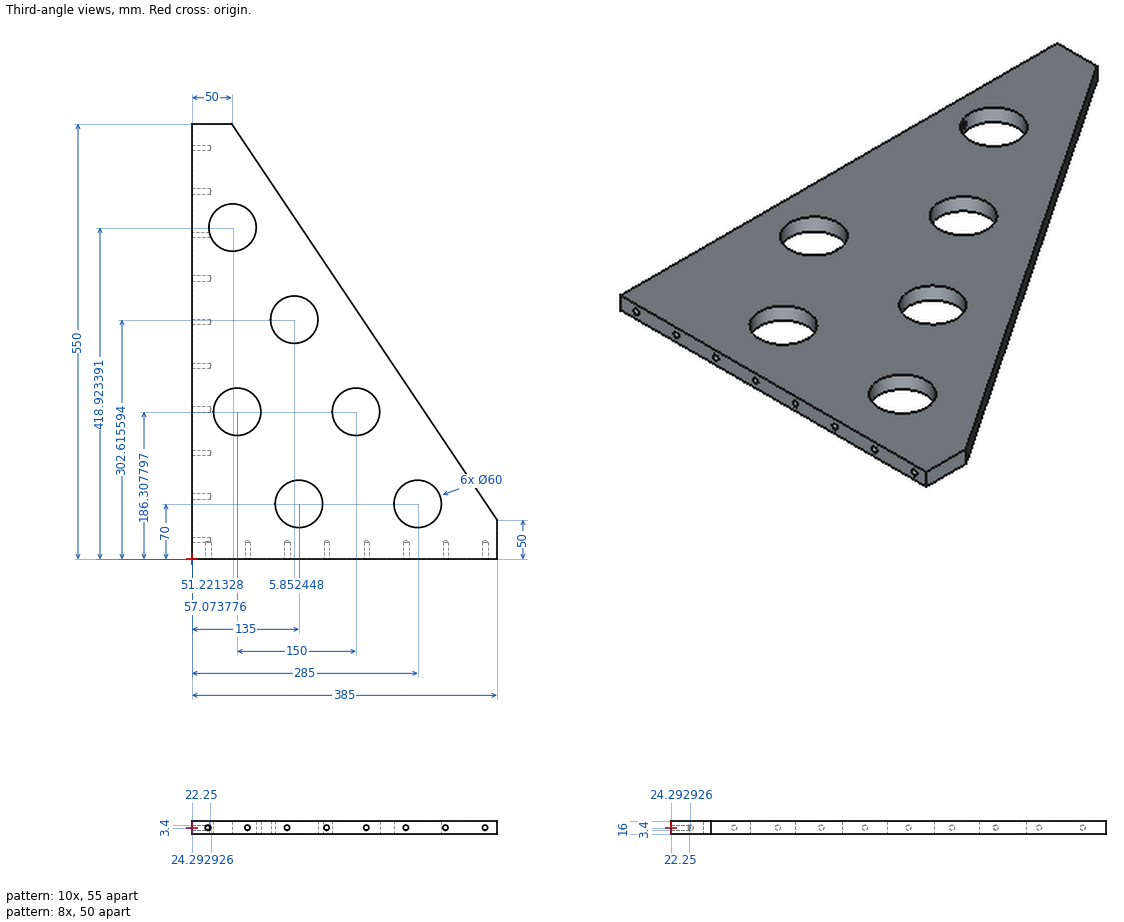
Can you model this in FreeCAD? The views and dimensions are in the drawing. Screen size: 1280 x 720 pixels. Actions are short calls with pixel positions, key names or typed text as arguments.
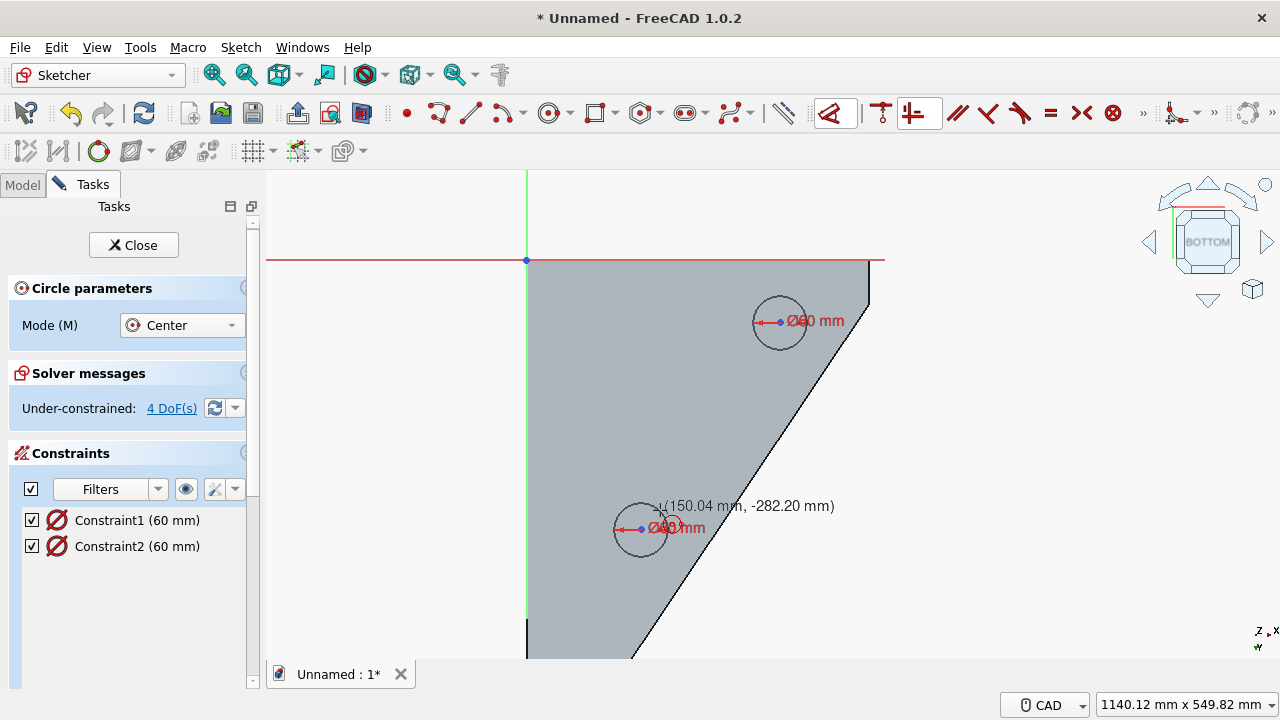
click(711, 426)
move(730, 407)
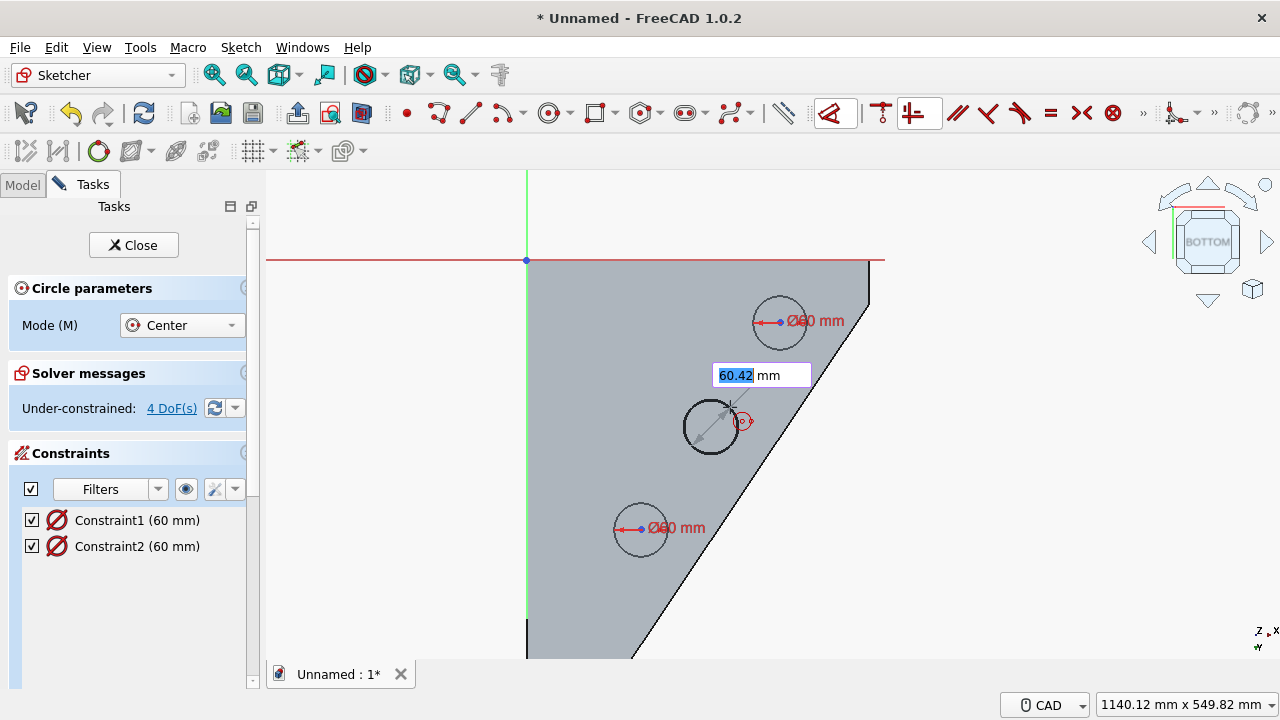
text(60)
key(Return)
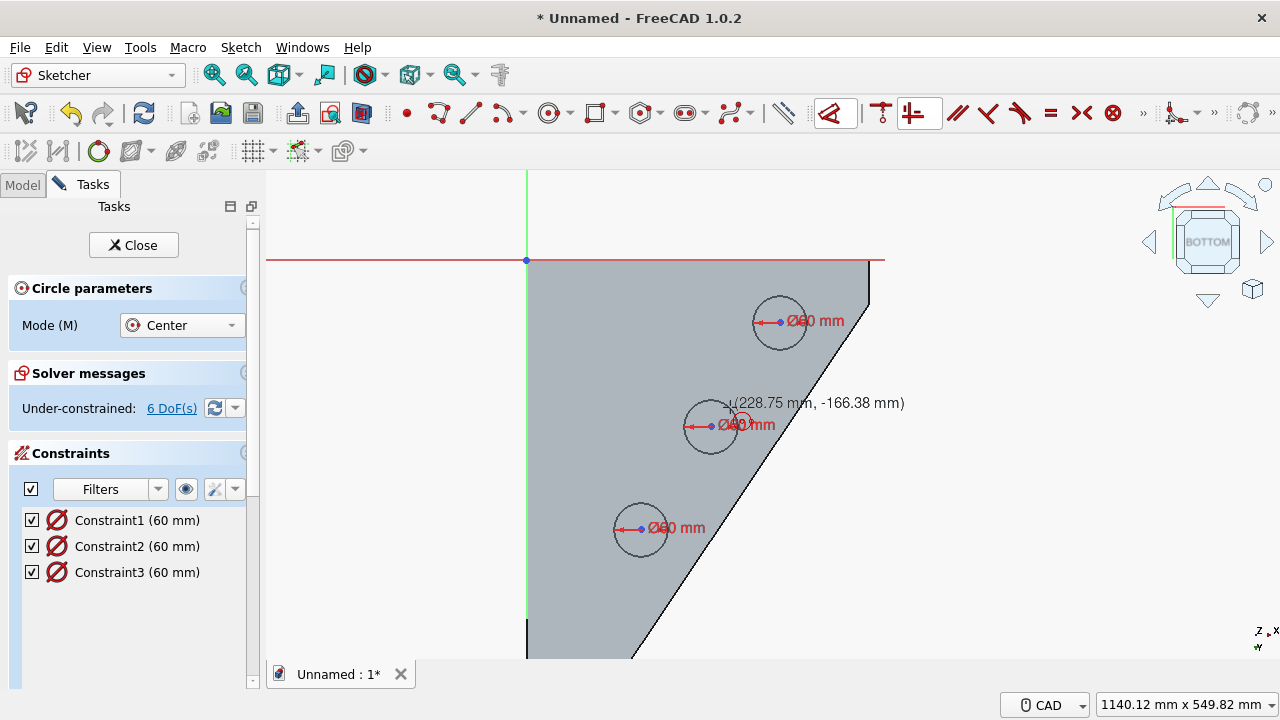
click(647, 322)
move(665, 303)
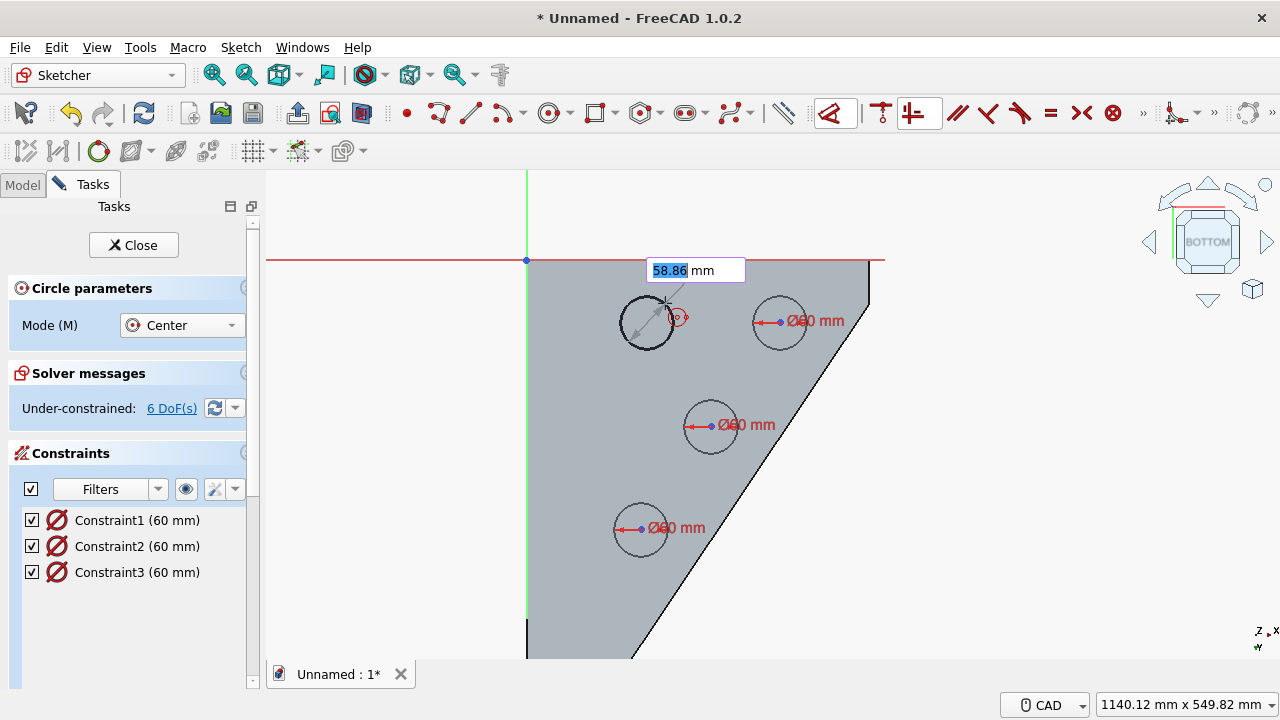
text(60)
key(Return)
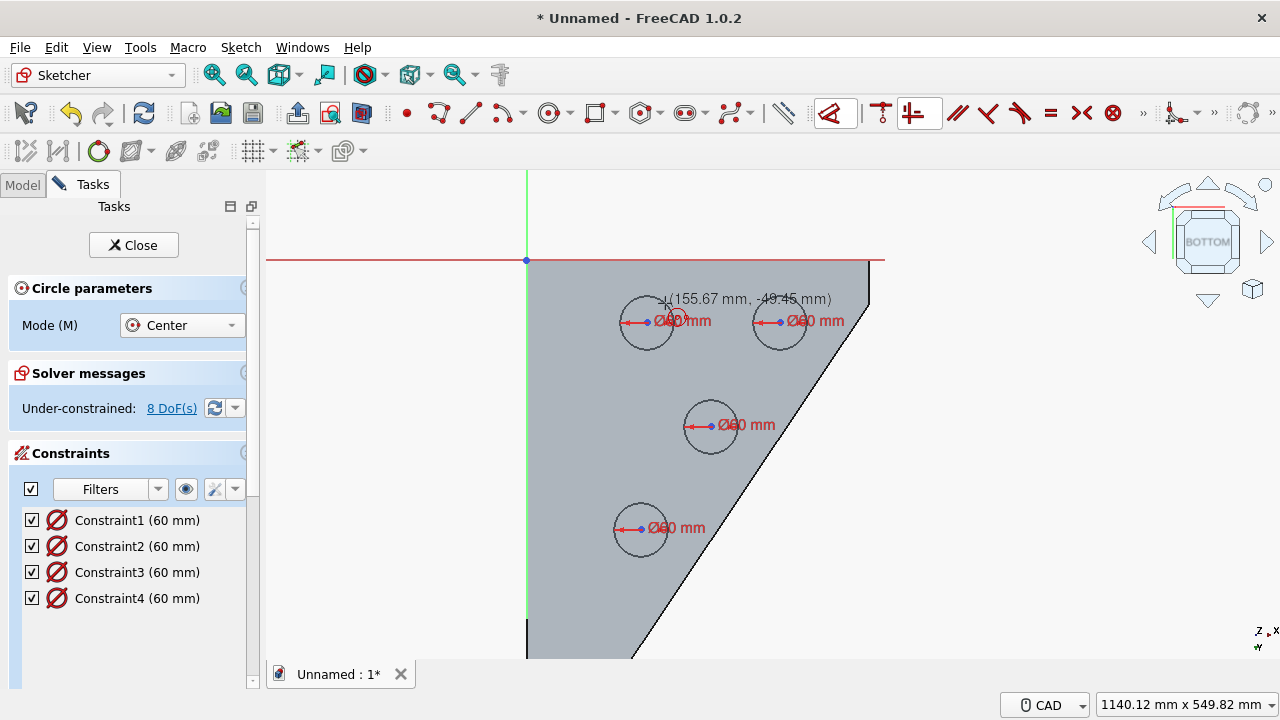
scroll(876, 211, down, 1)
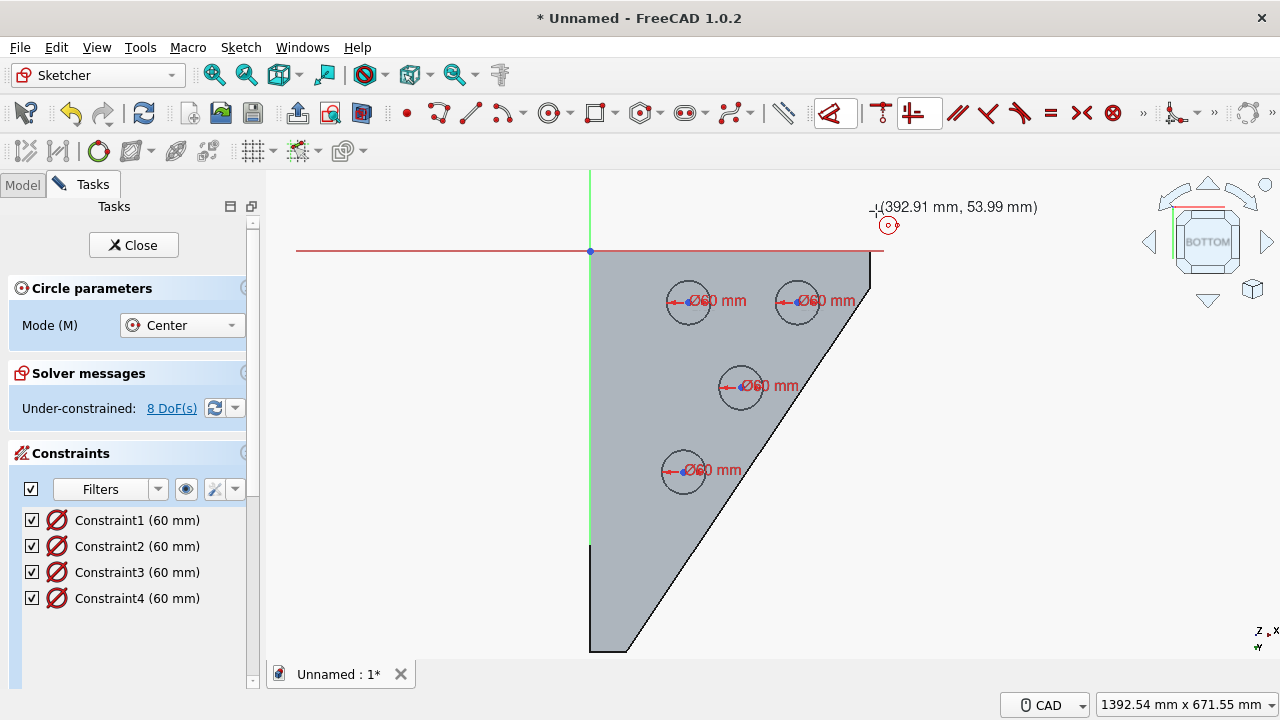
click(627, 556)
move(643, 541)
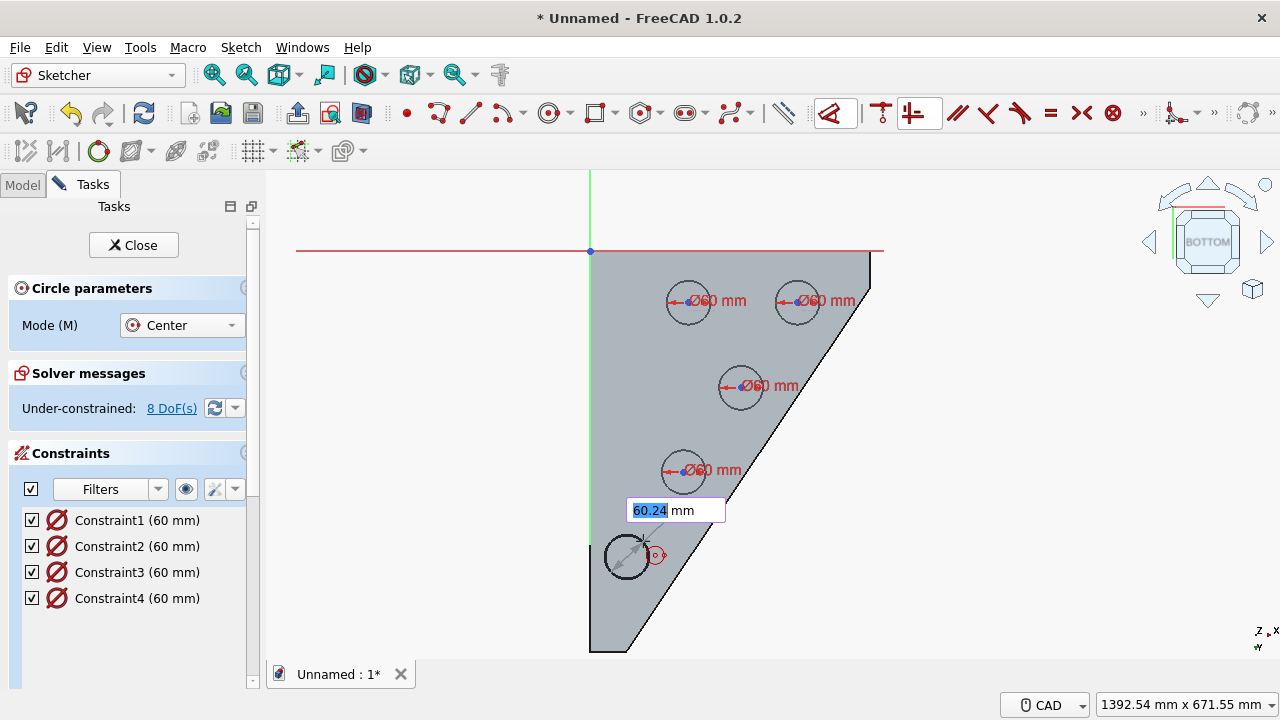
text(60)
key(Return)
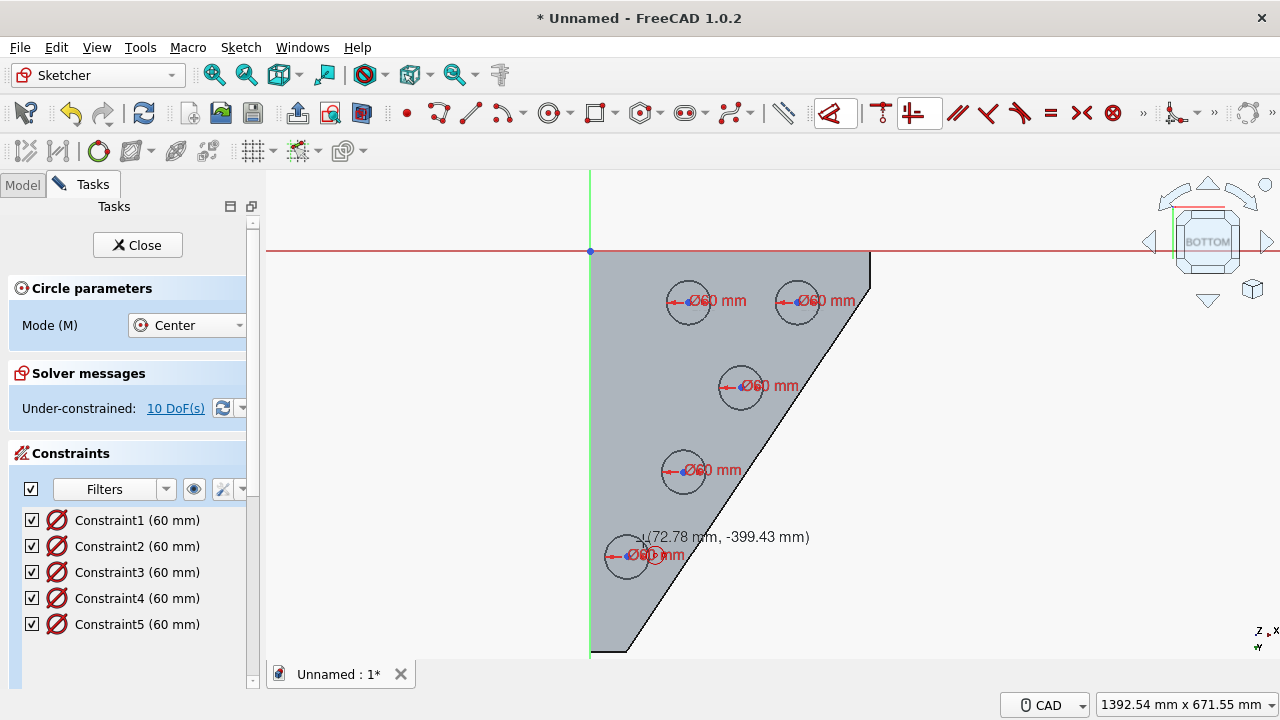
click(632, 387)
move(647, 371)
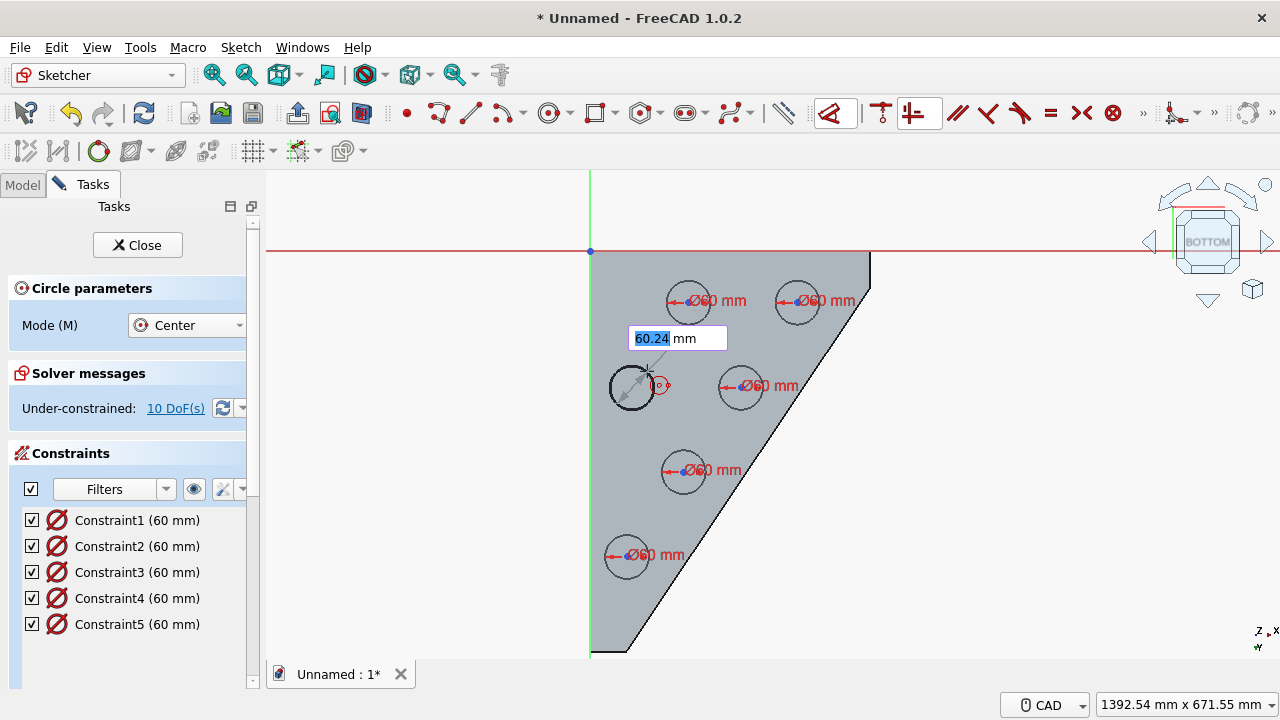
text(60)
key(Return)
key(Escape)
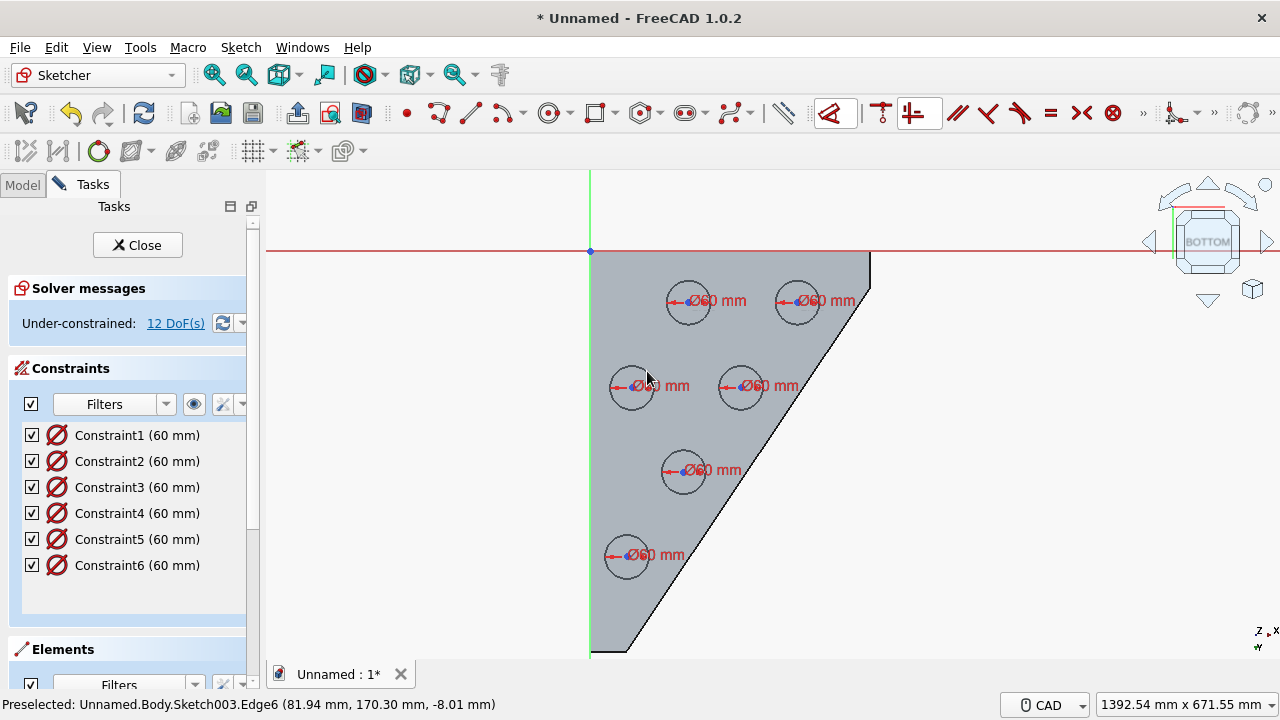
click(798, 303)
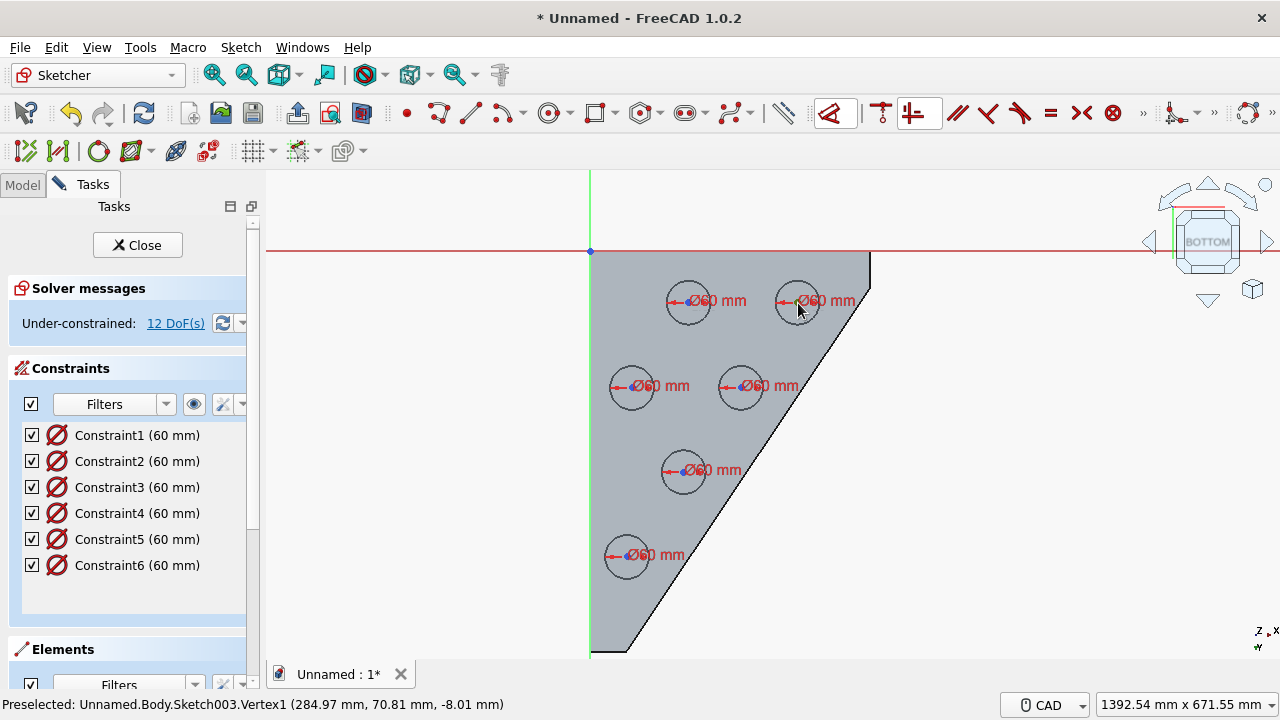
click(689, 303)